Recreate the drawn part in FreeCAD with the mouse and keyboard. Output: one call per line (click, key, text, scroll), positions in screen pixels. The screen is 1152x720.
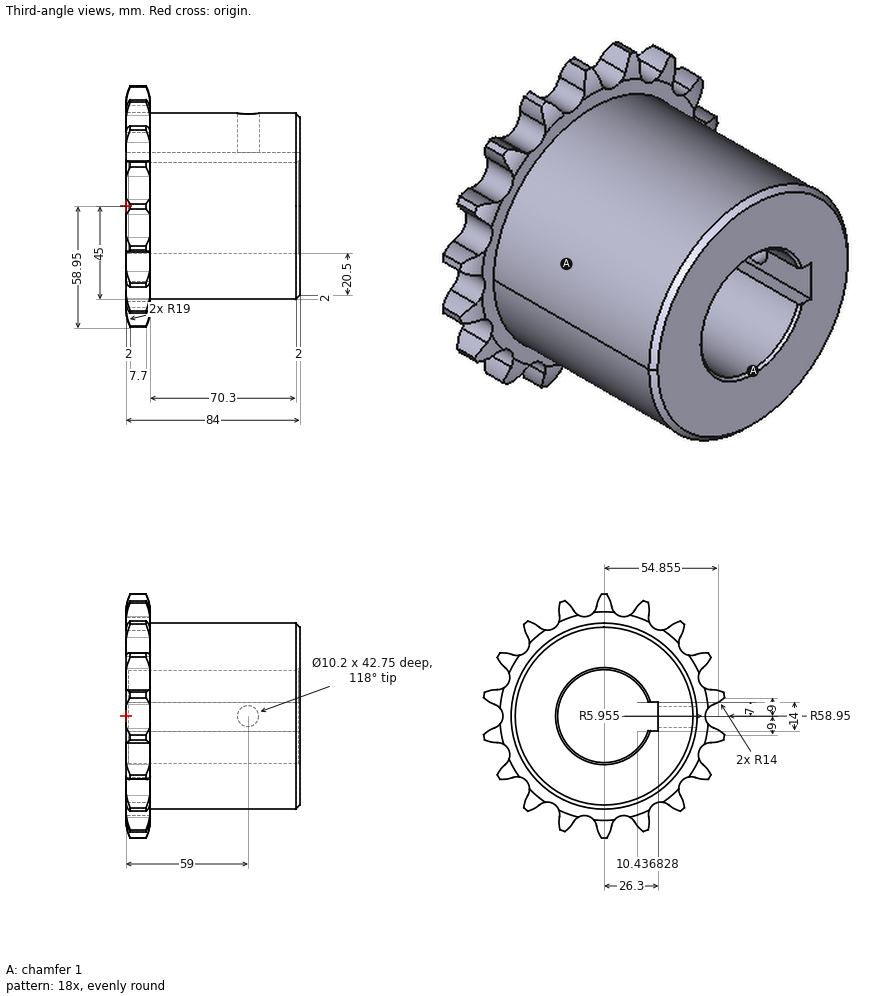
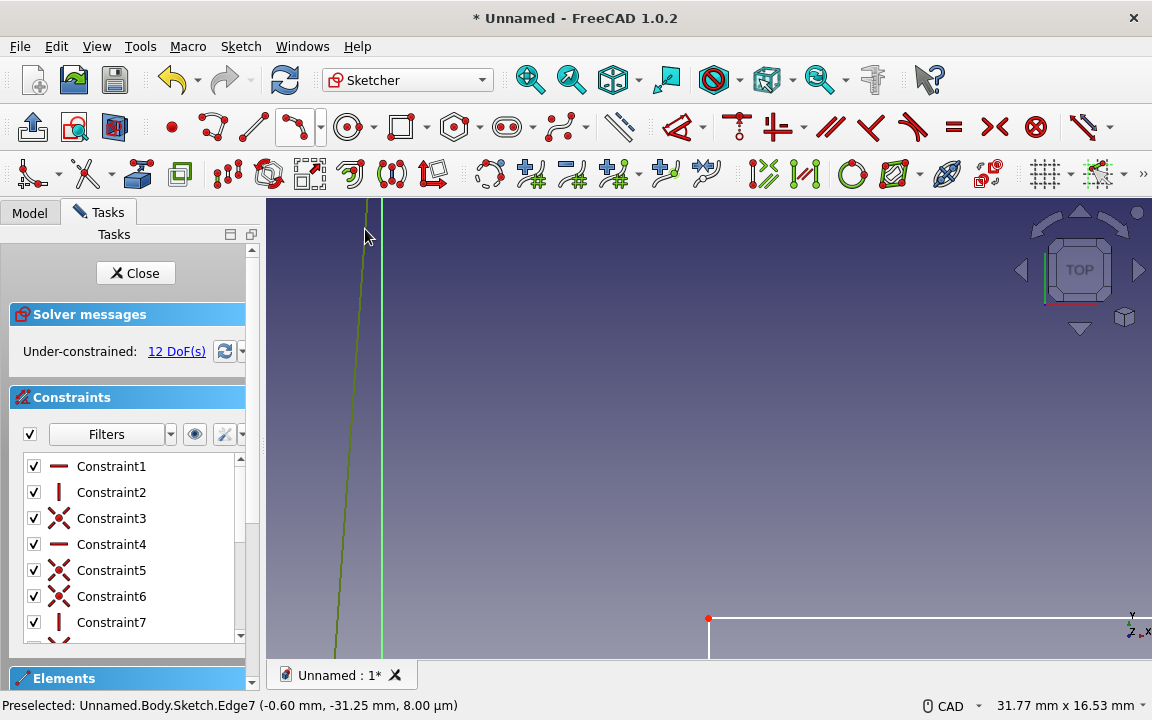
key(v)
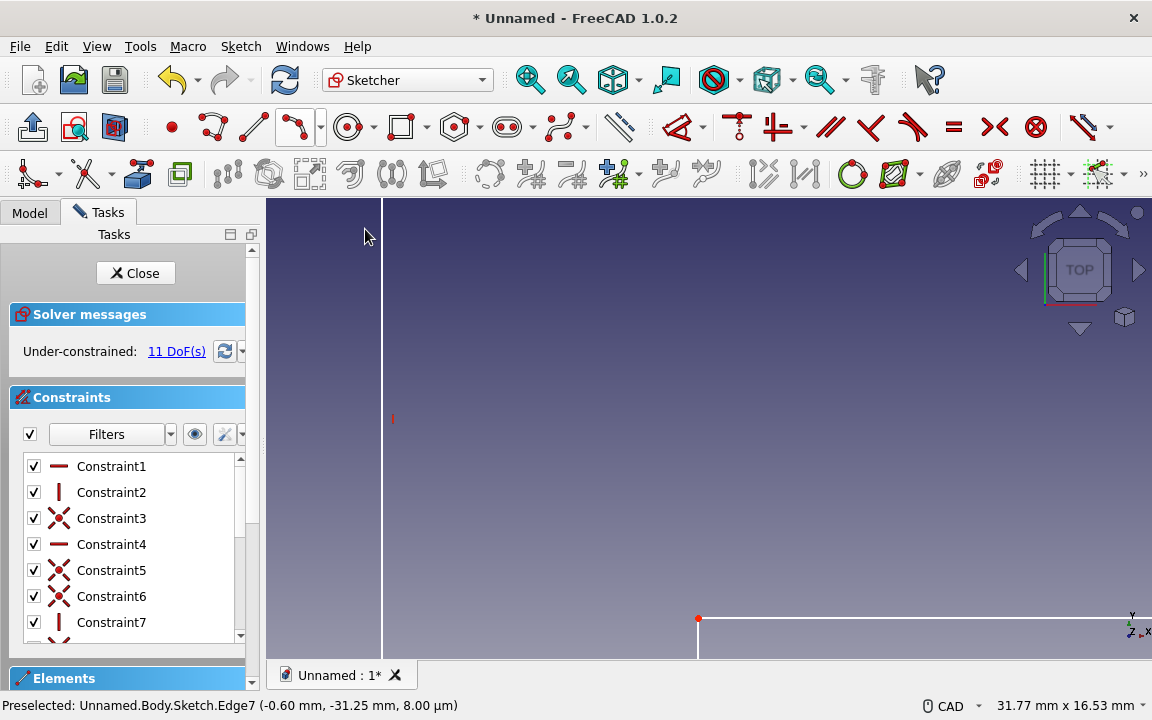
scroll(460, 478, down, 9)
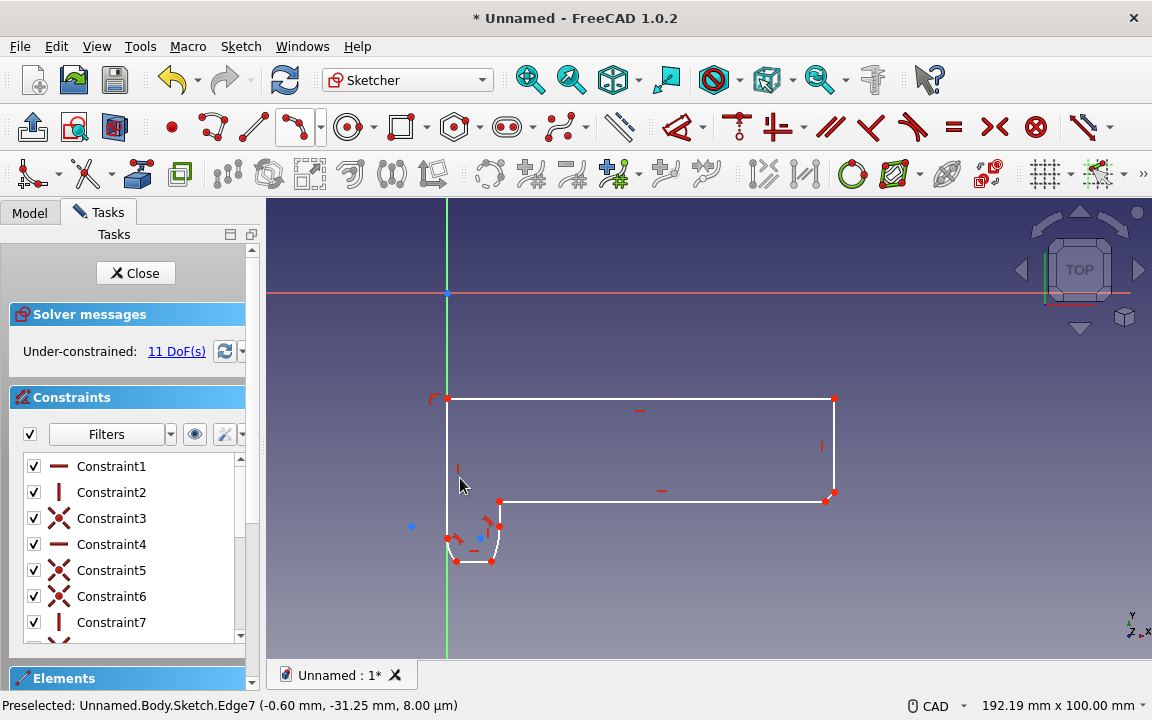
scroll(496, 552, up, 2)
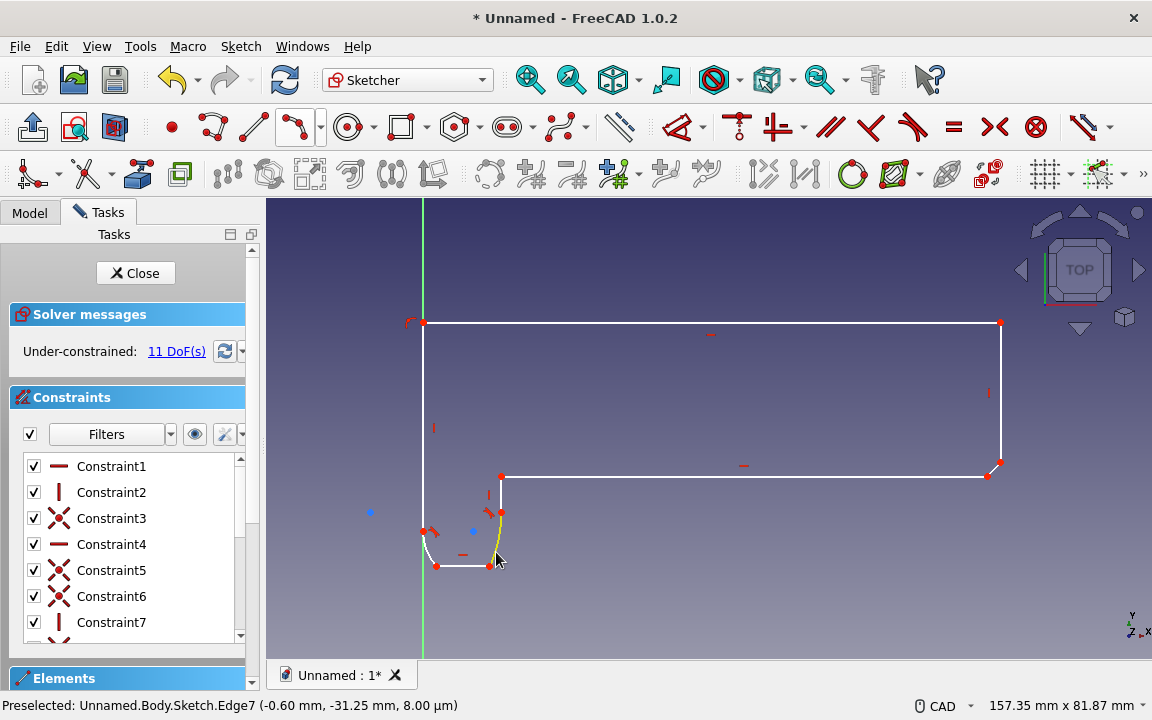
click(496, 551)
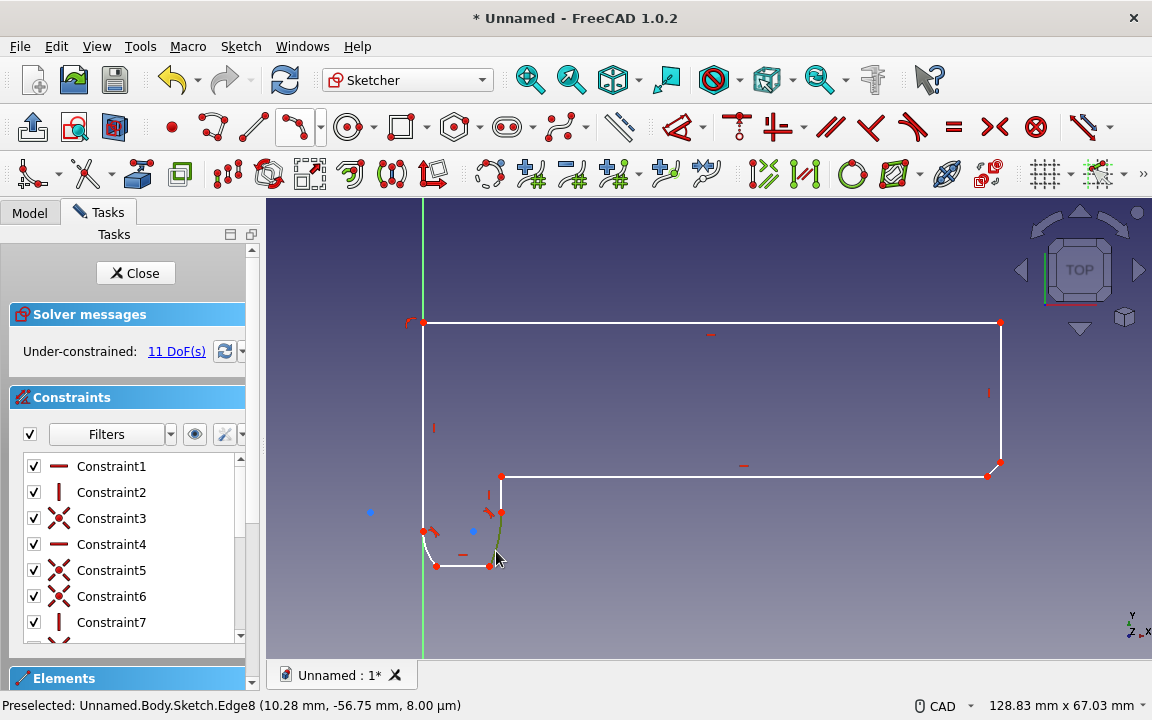
click(425, 543)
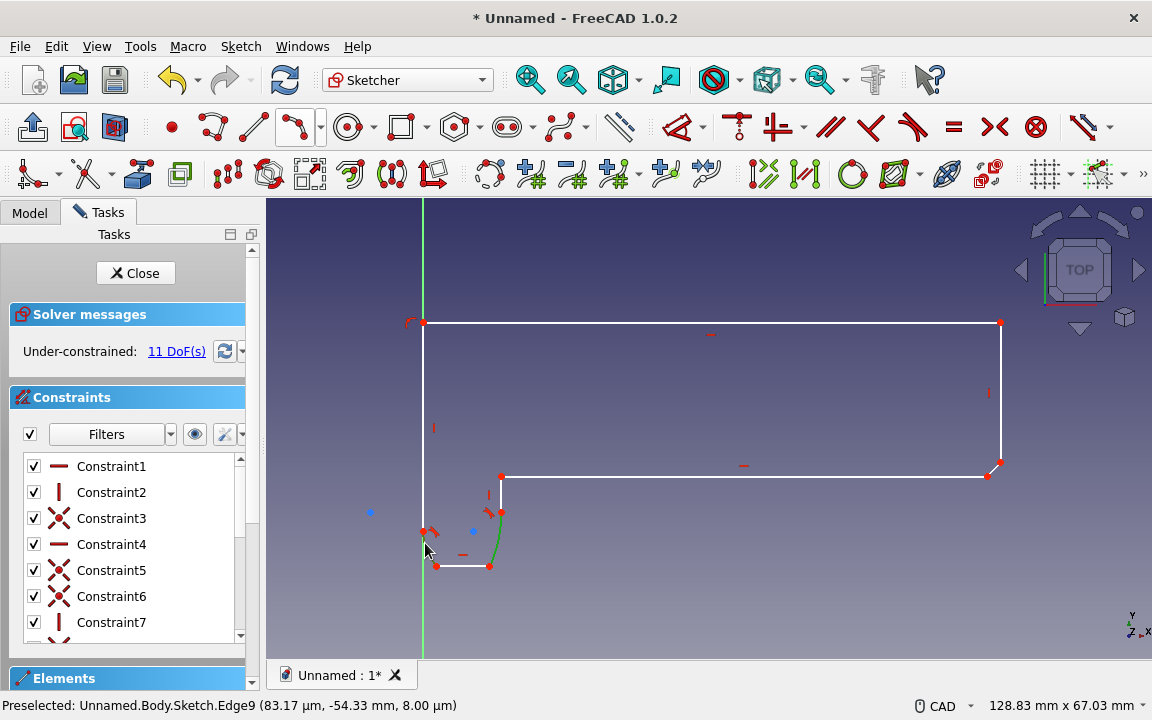
click(954, 128)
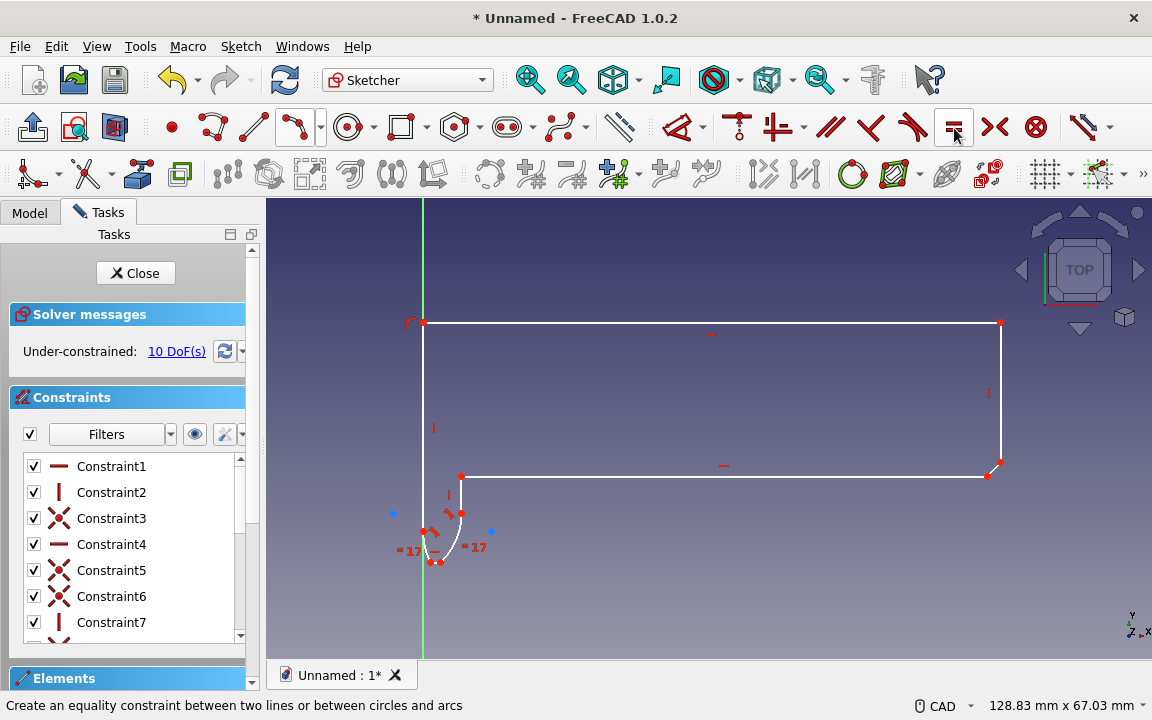
click(676, 128)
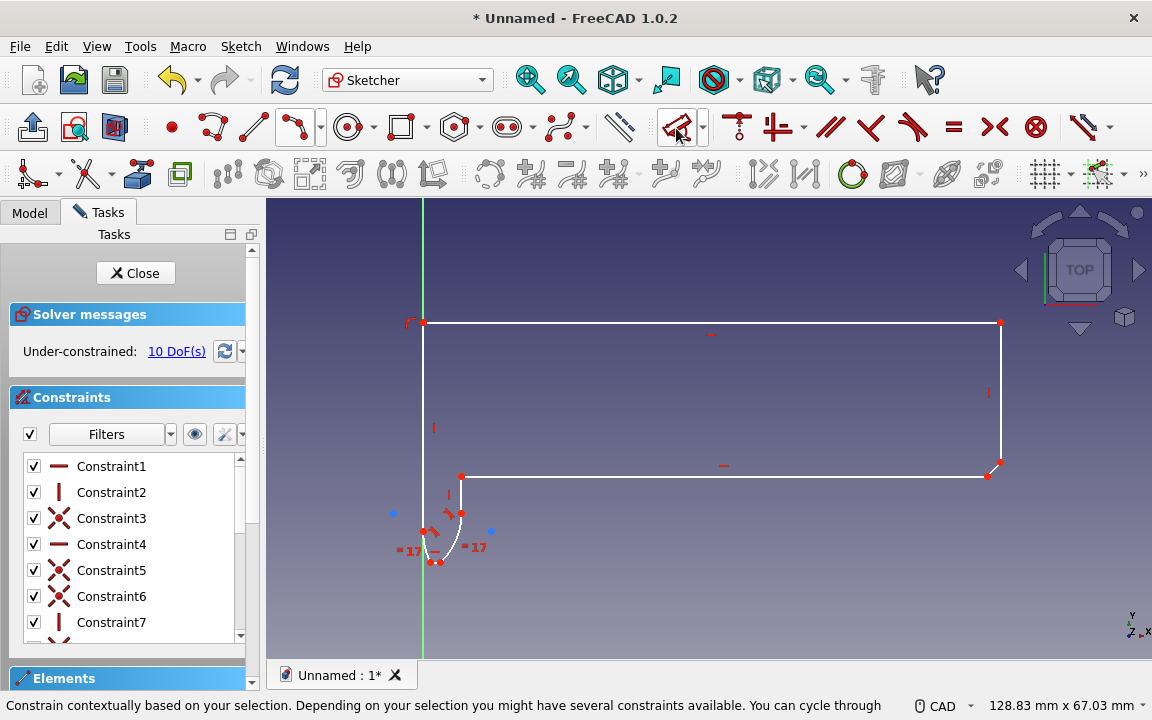
click(451, 550)
click(478, 567)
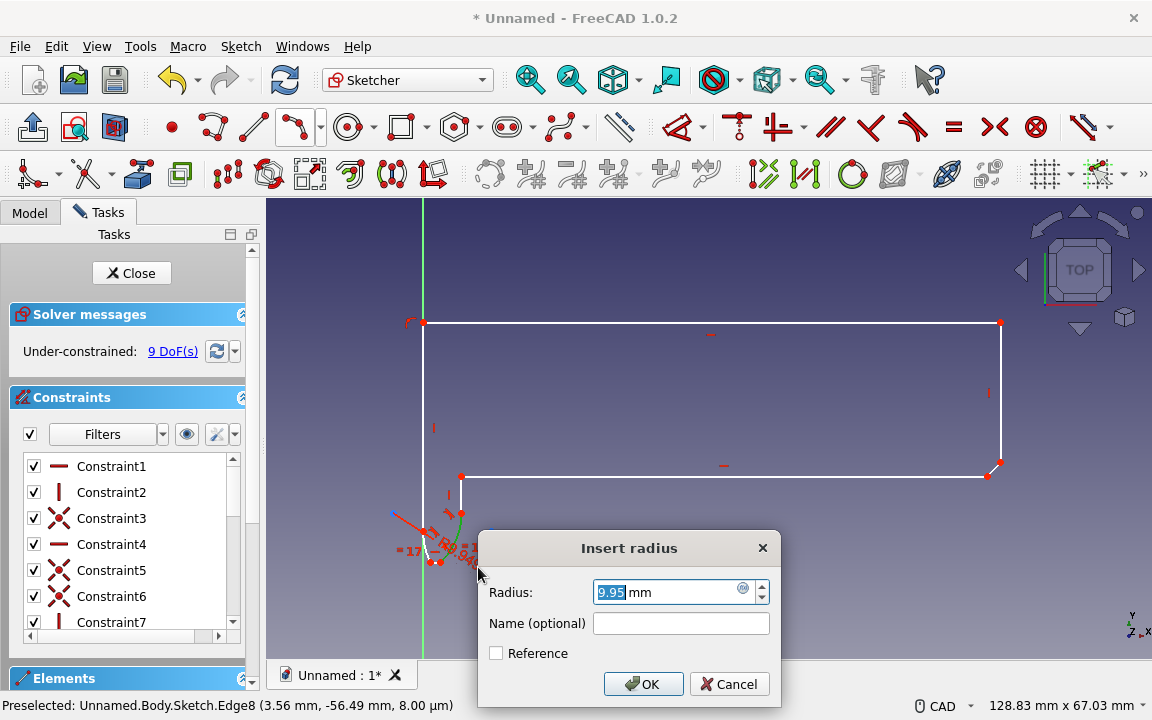
text(19)
key(Return)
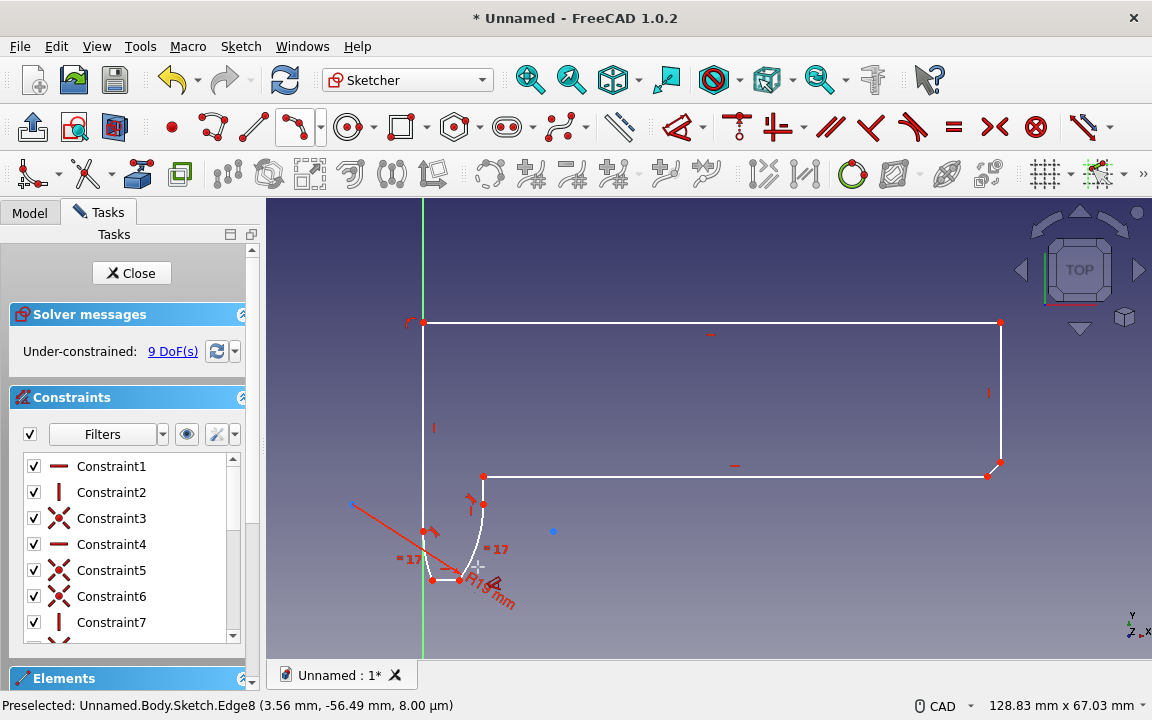
click(827, 323)
click(705, 289)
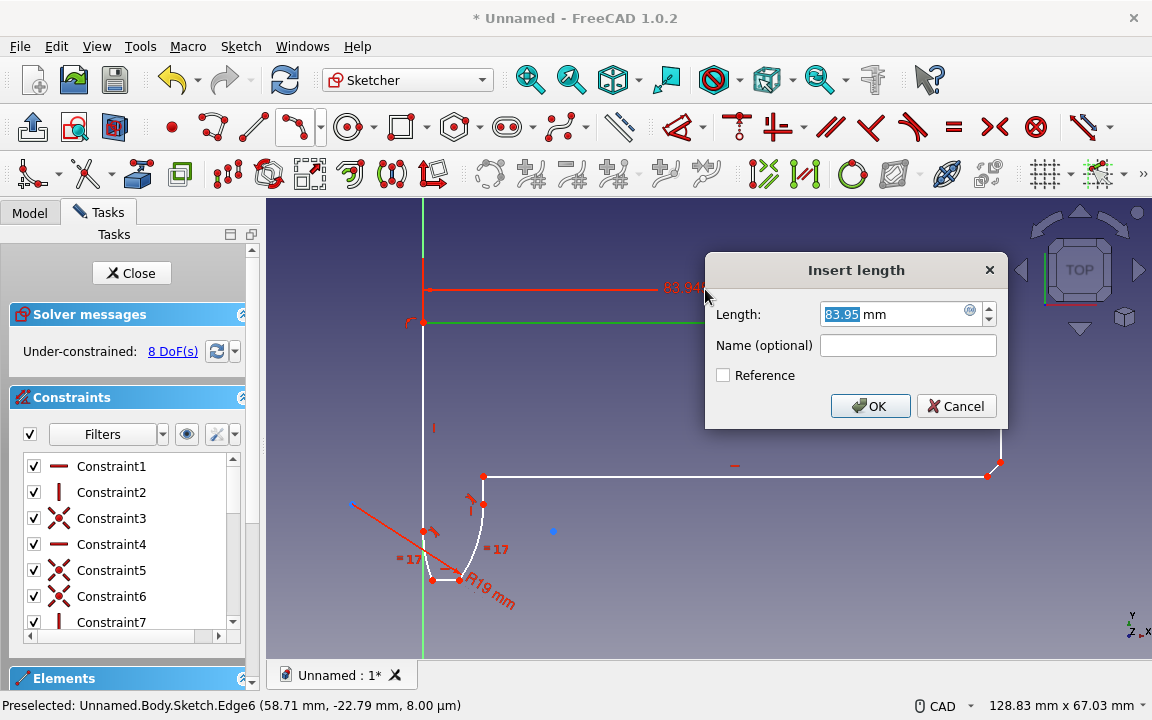
text(84)
key(Return)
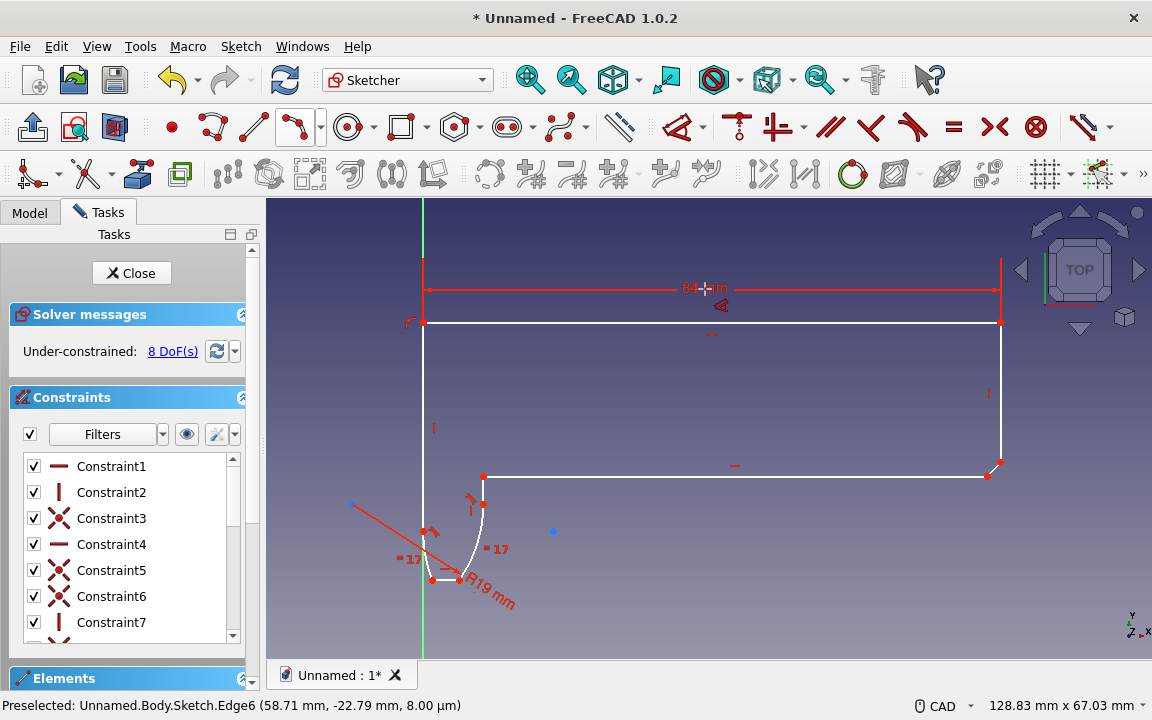
scroll(432, 580, up, 6)